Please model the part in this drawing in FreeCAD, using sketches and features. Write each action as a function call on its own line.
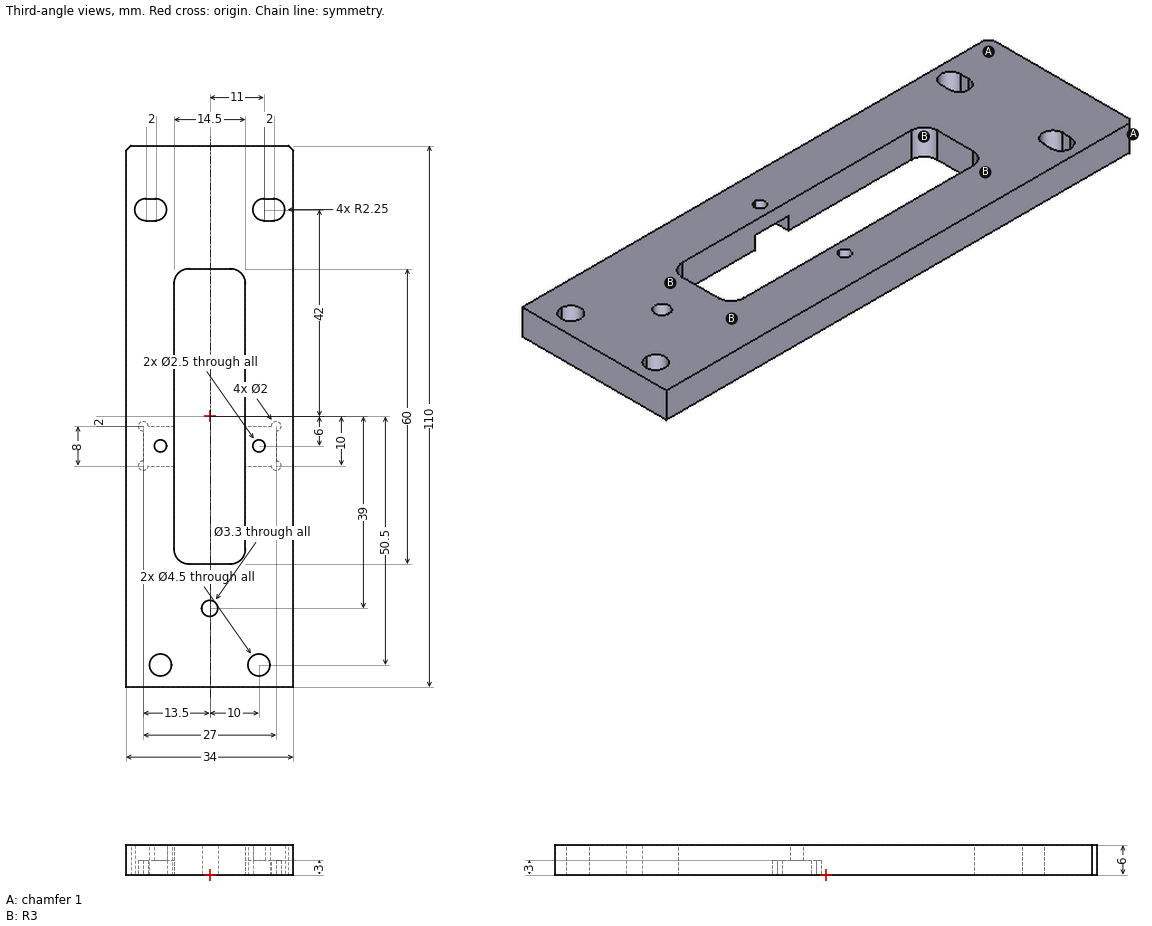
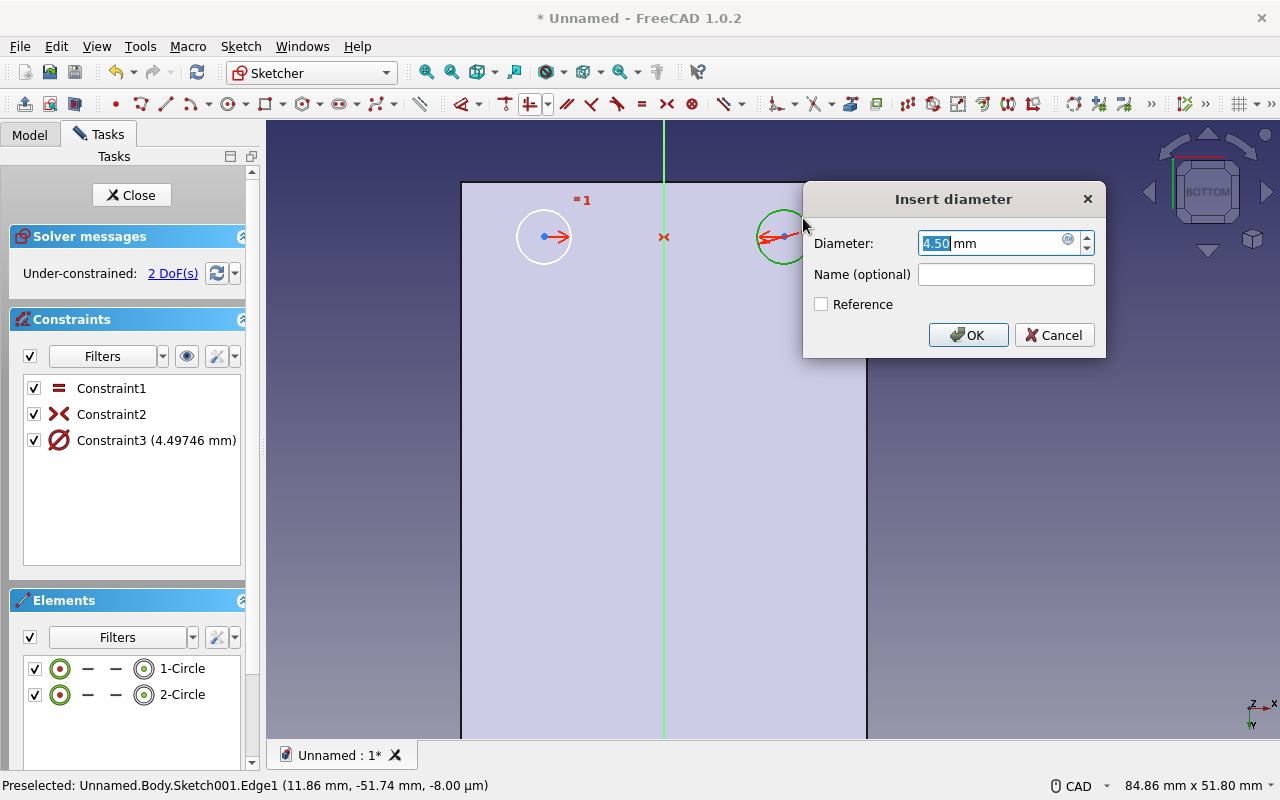
text(4.5)
key(Return)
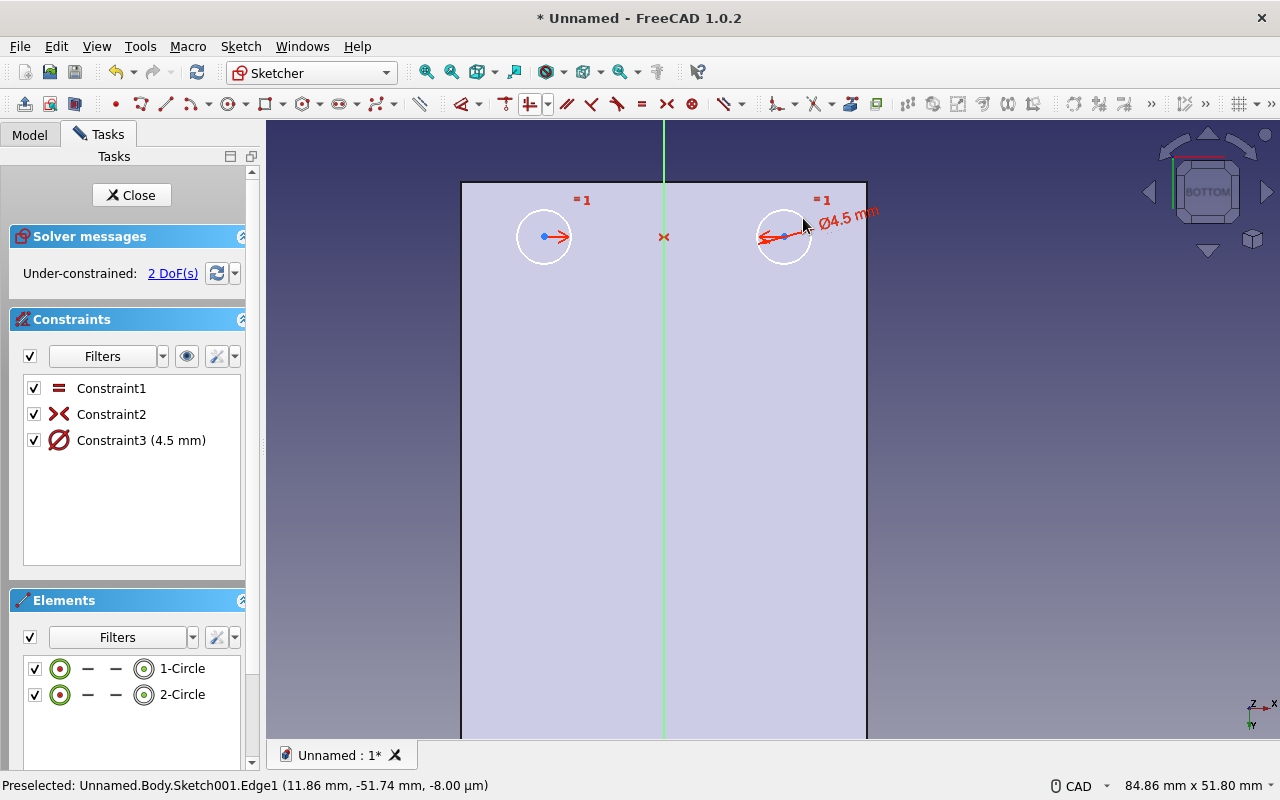
click(784, 237)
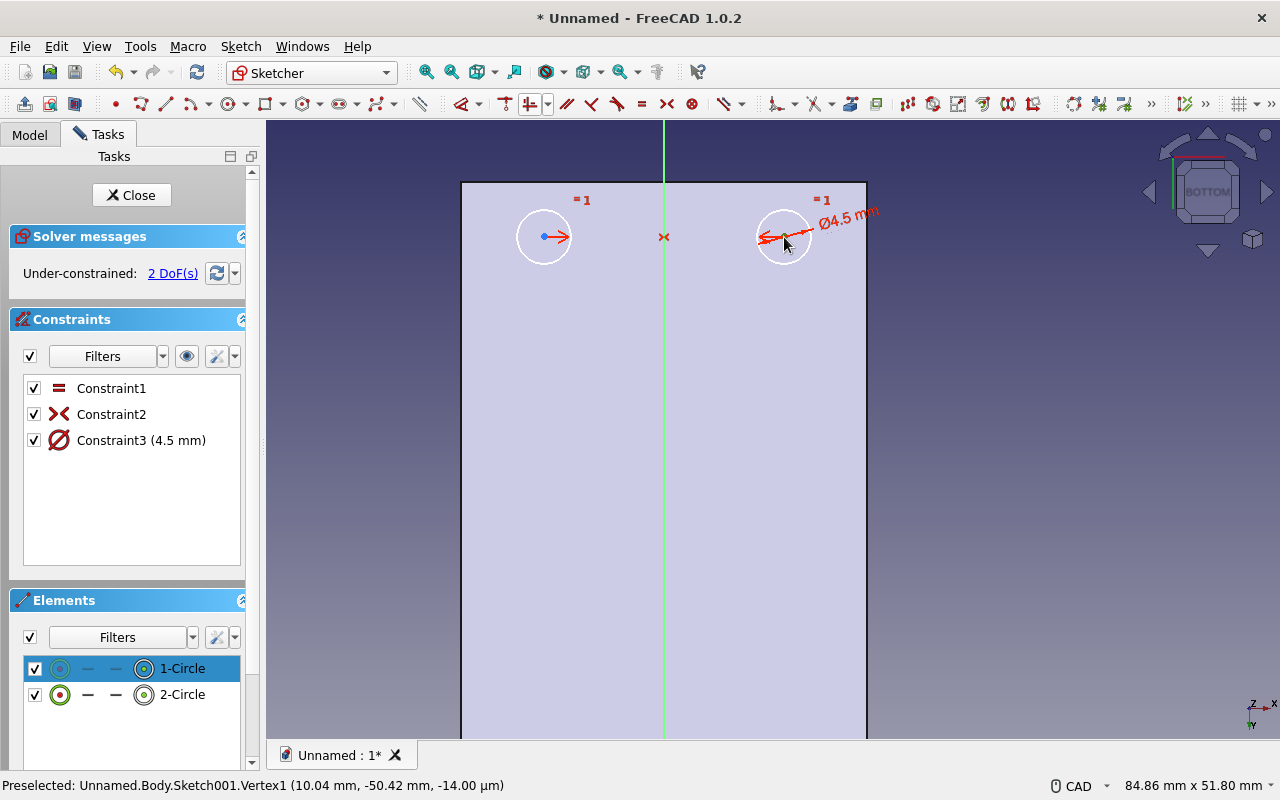
key(l)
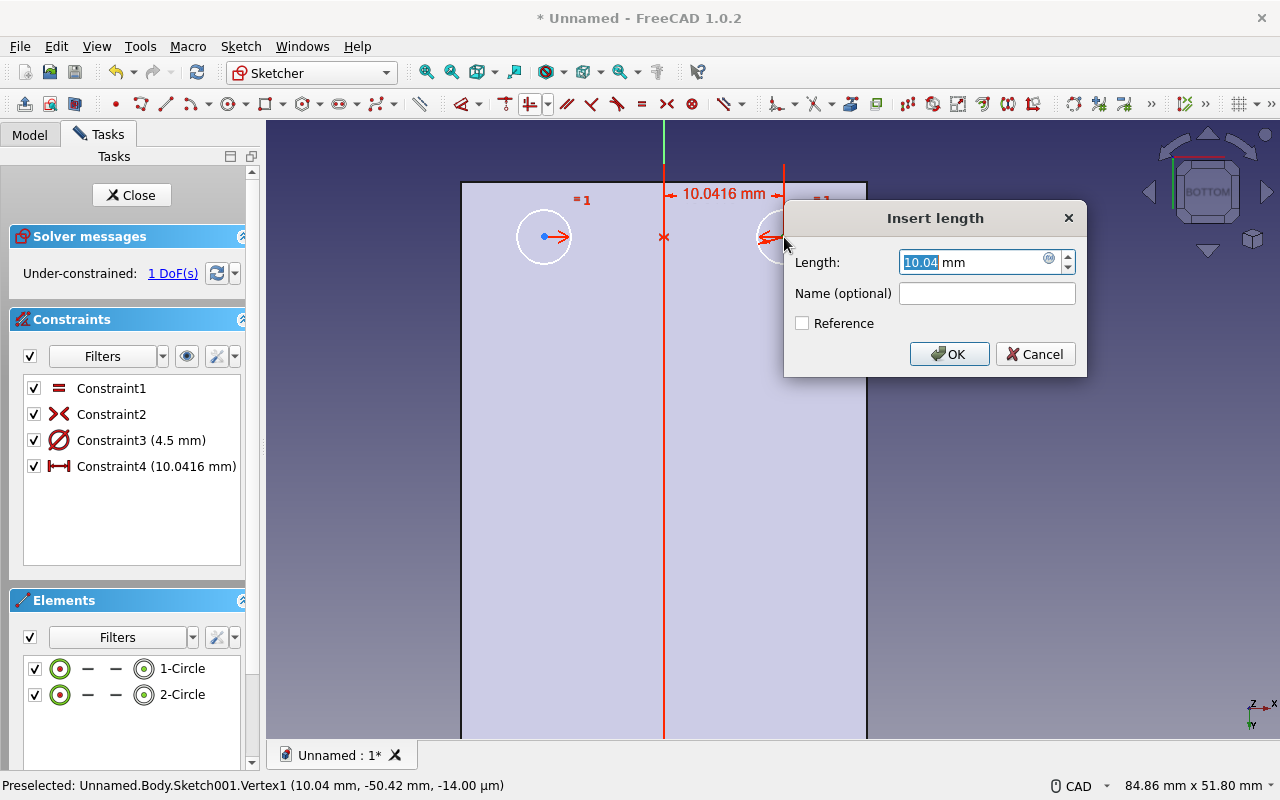
text(10)
key(Return)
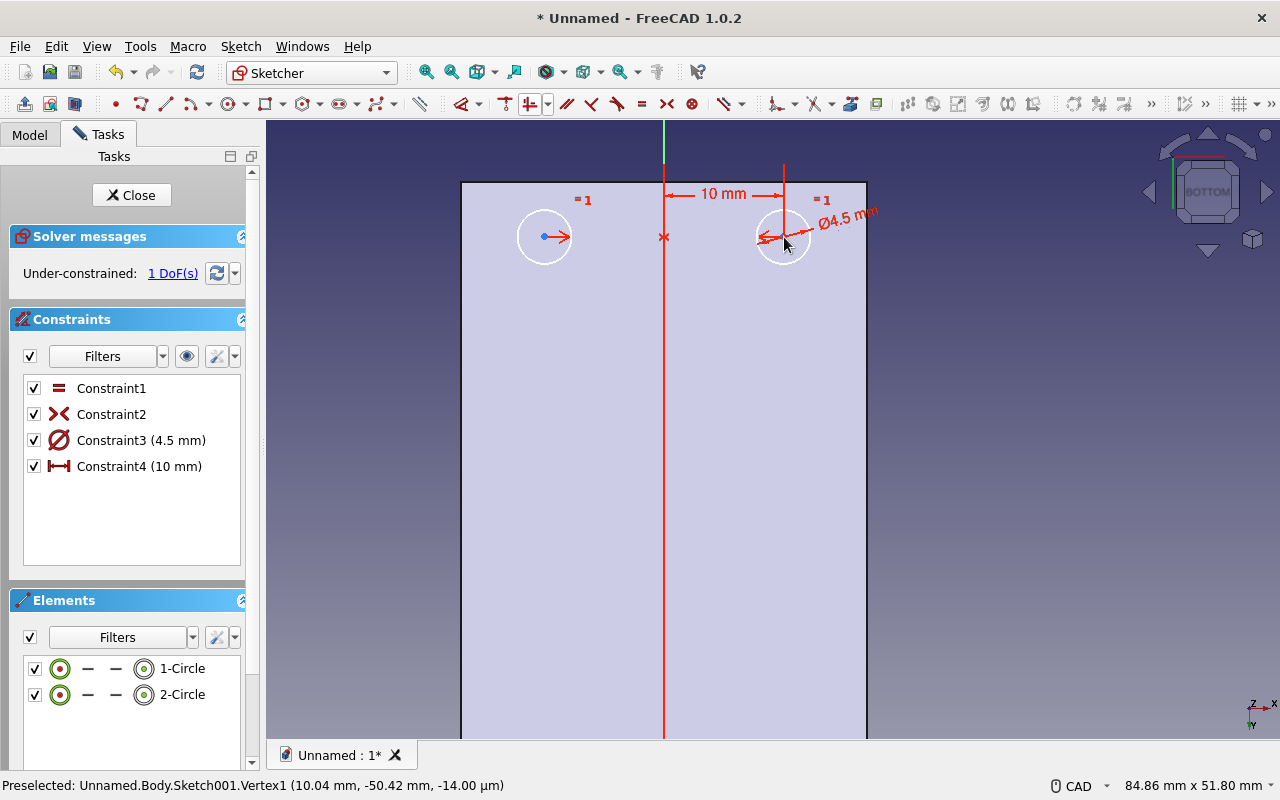
click(784, 237)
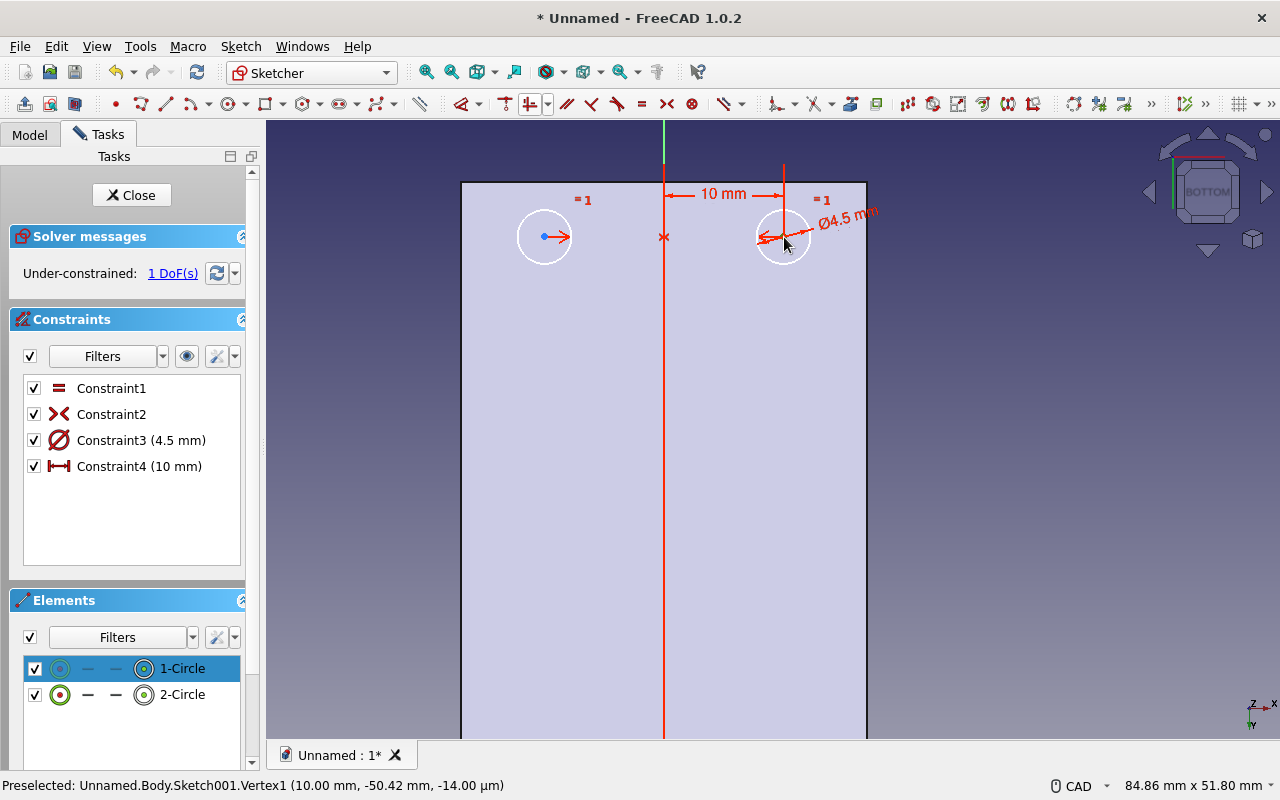
key(i)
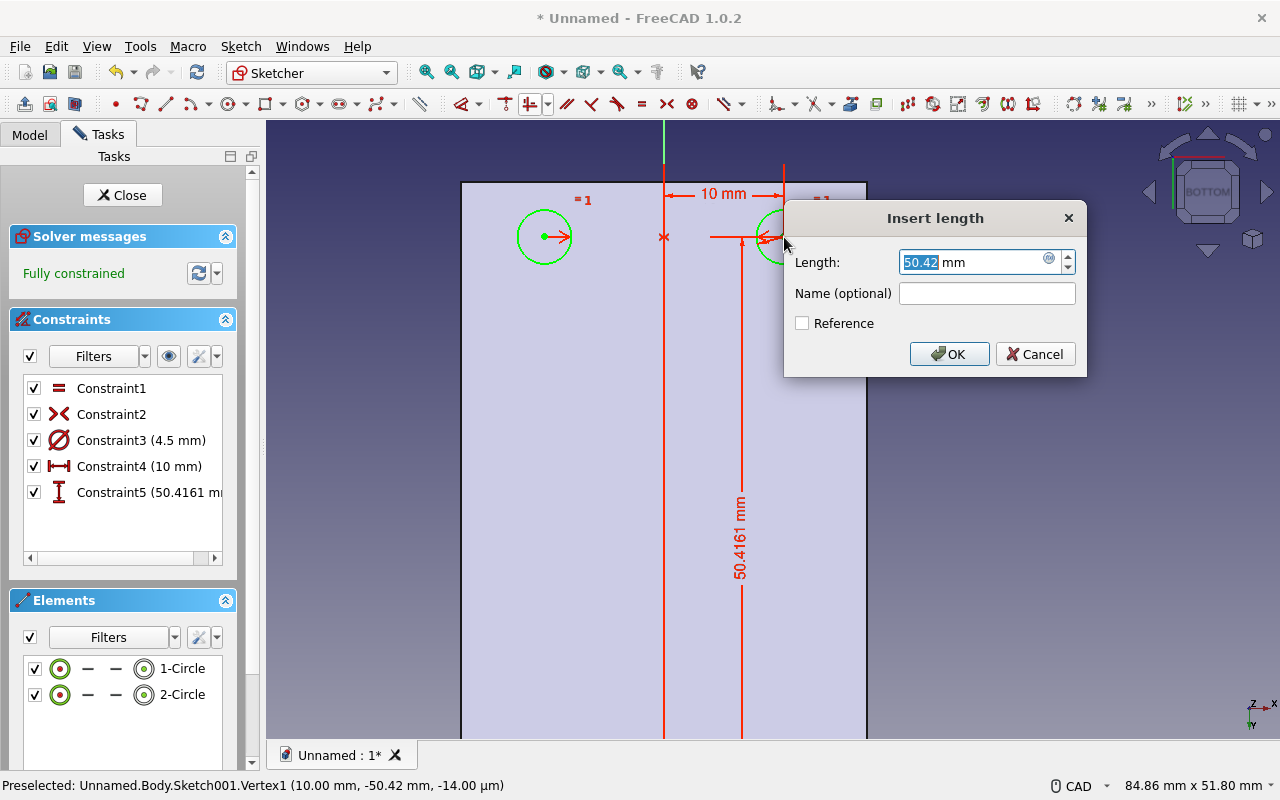
text(50.5)
key(Return)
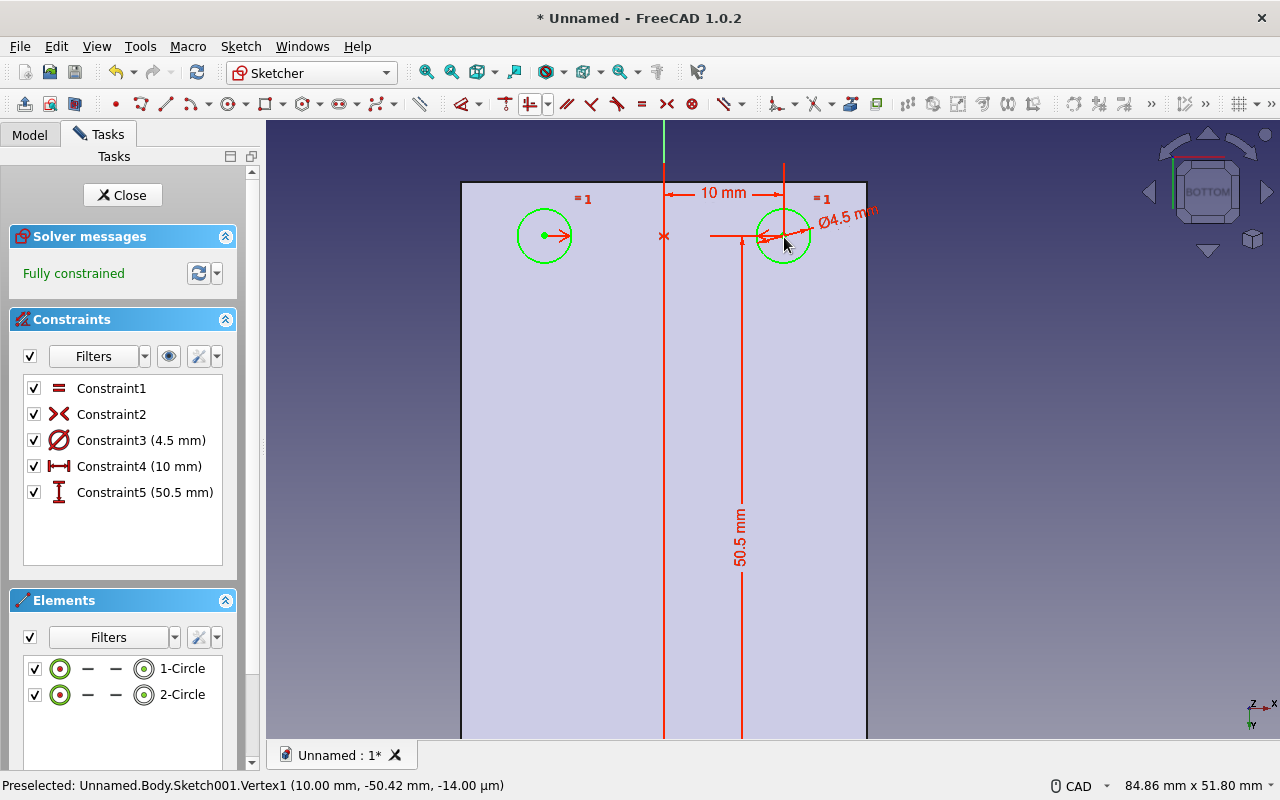
click(123, 195)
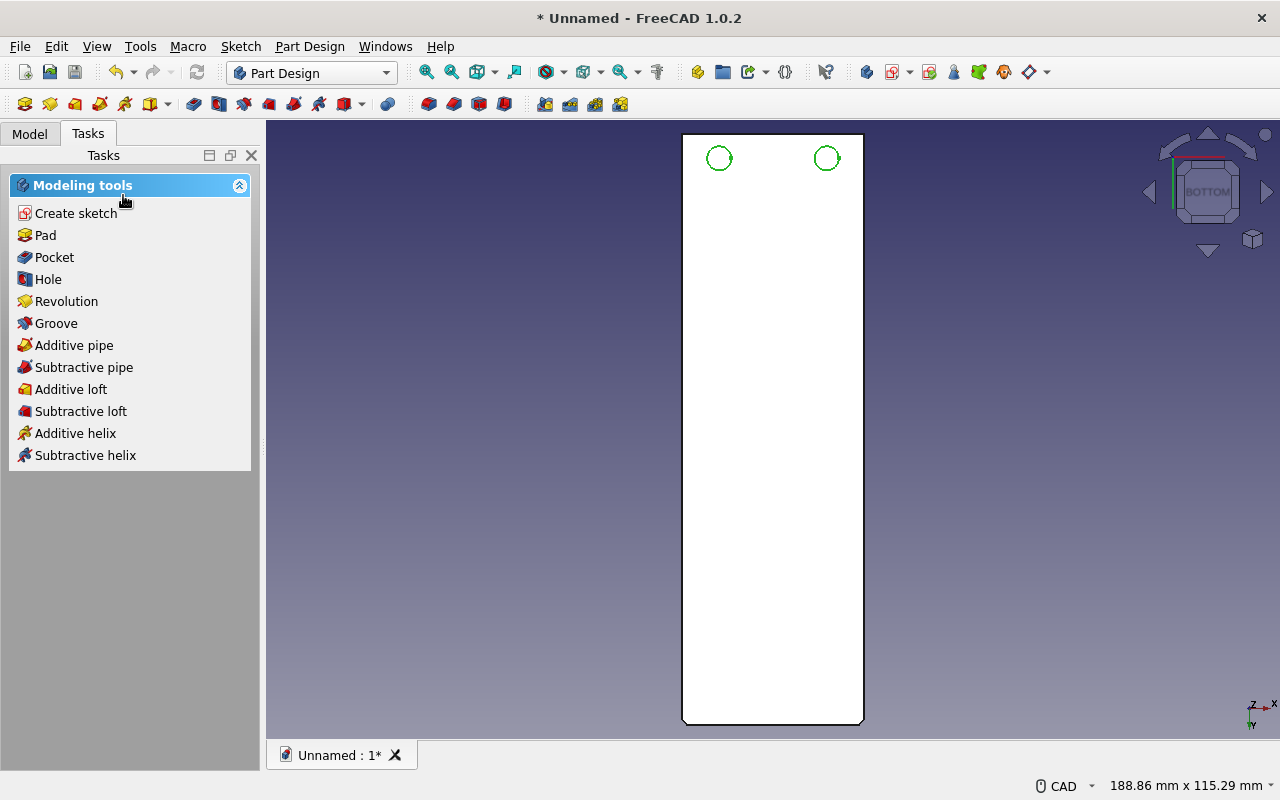
click(219, 104)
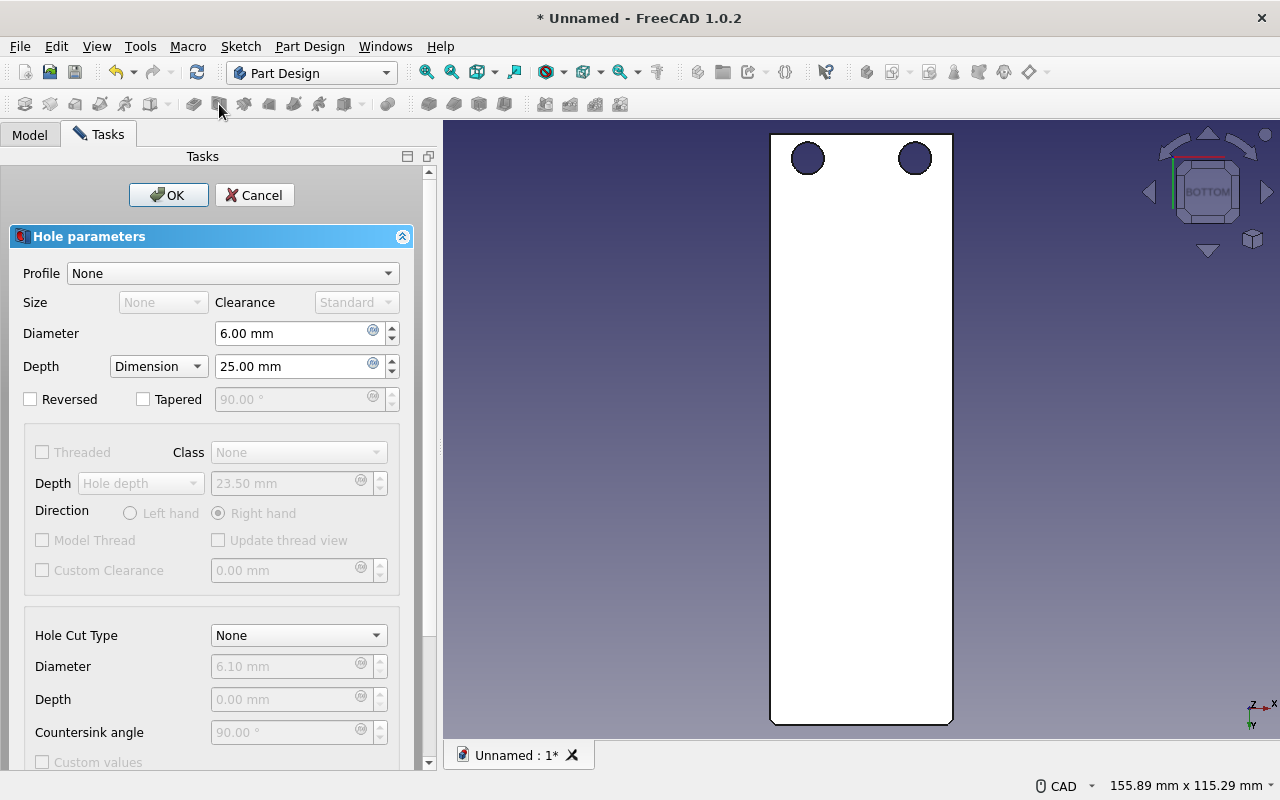
triple_click(300, 334)